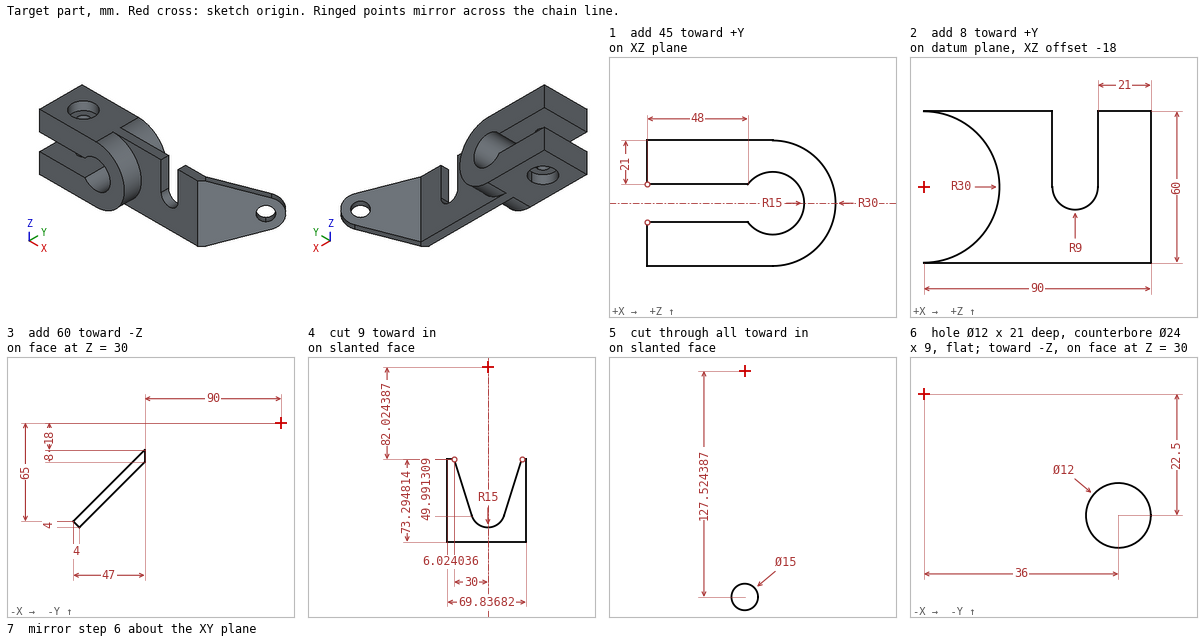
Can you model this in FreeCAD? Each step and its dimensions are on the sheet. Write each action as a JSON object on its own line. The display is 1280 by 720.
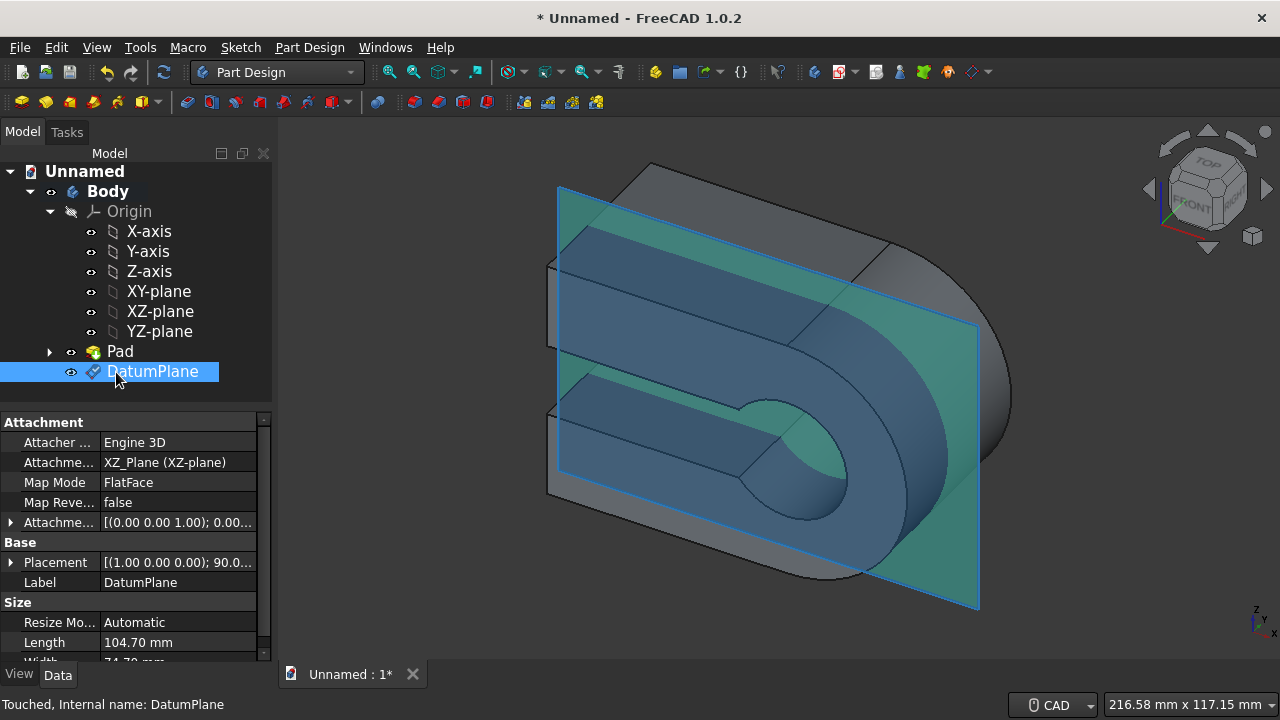
{"action": "left_click", "coordinate": [840, 72]}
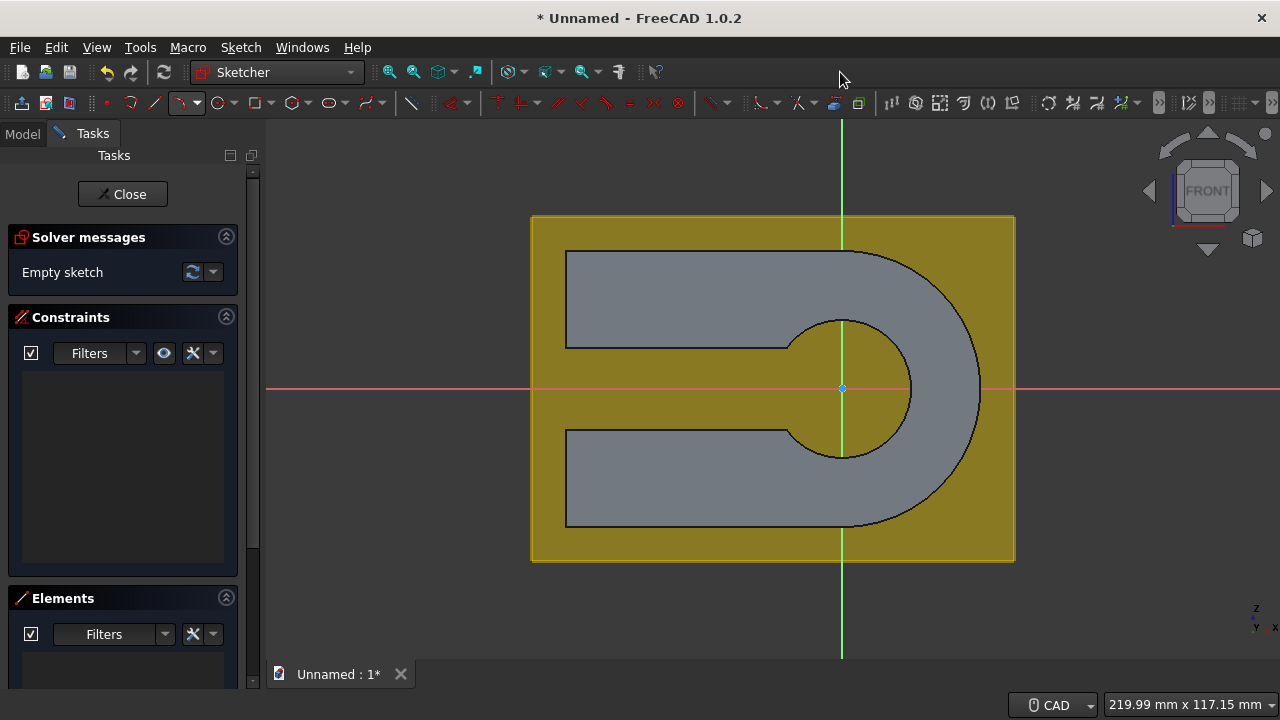
{"action": "left_click", "coordinate": [70, 104]}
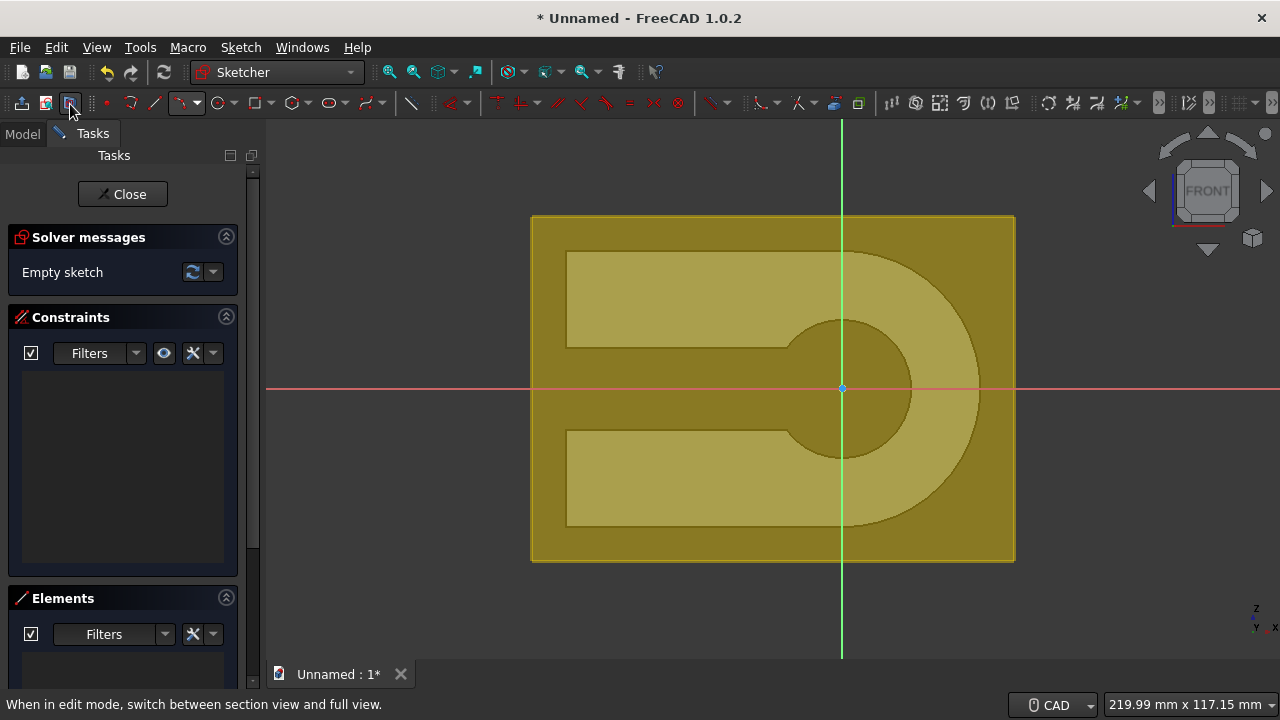
{"action": "scroll", "coordinate": [294, 389], "scroll_direction": "down", "scroll_amount": 1}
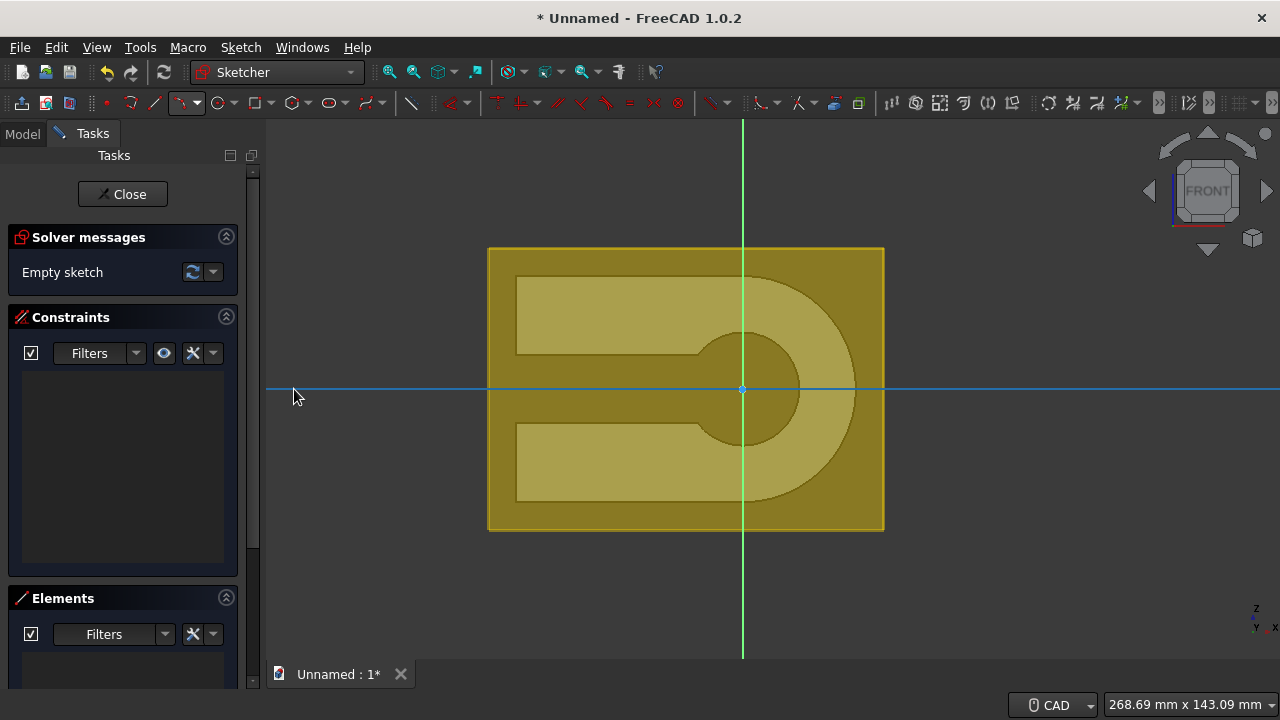
{"action": "scroll", "coordinate": [1115, 389], "scroll_direction": "up", "scroll_amount": 2}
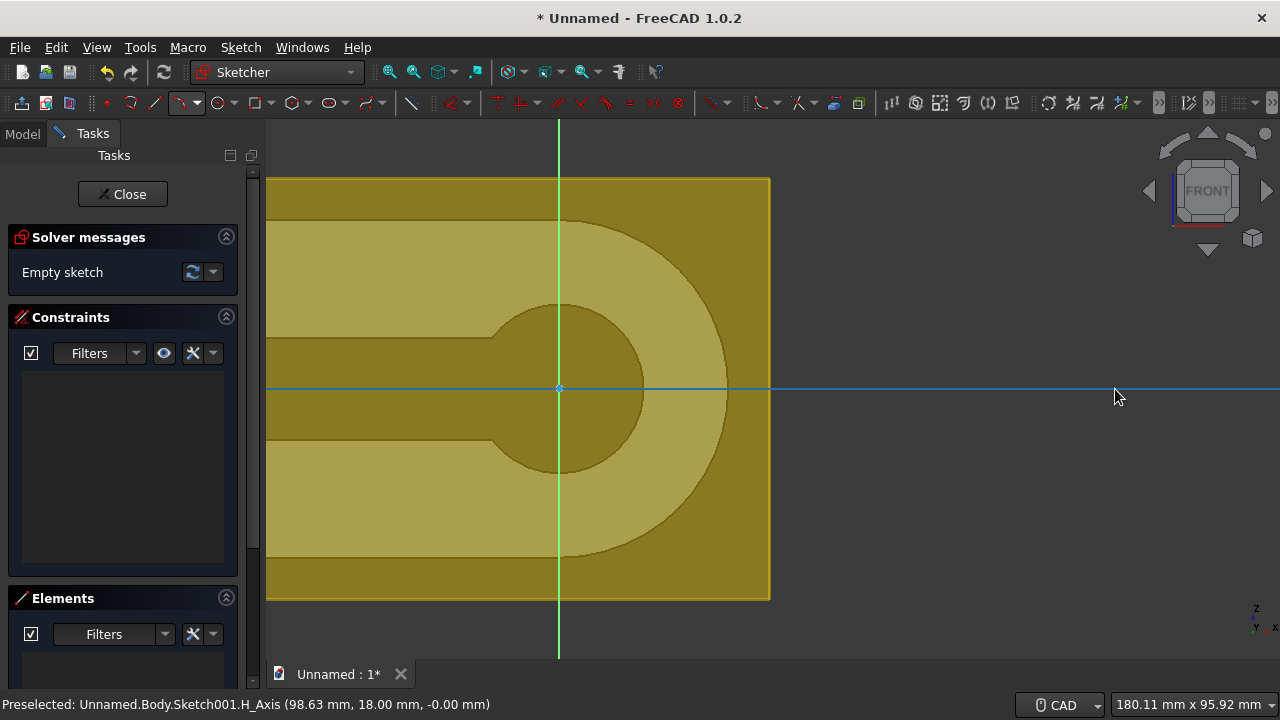
{"action": "left_click", "coordinate": [132, 104]}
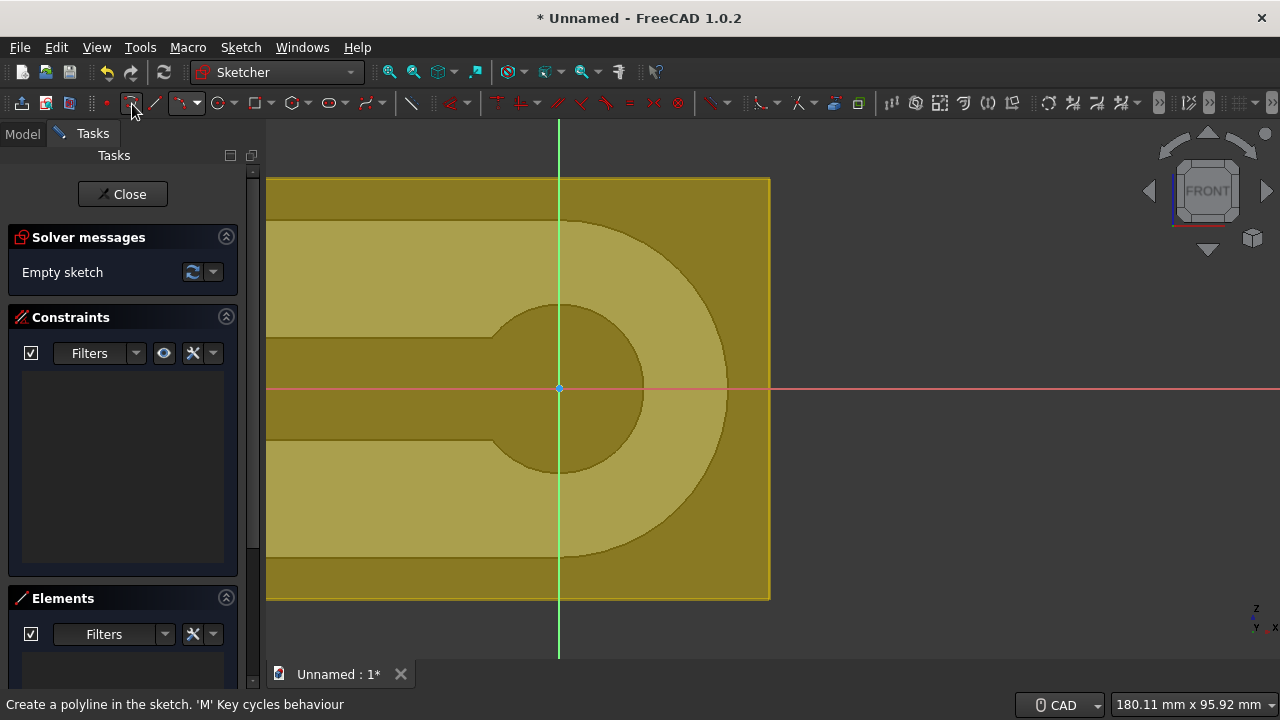
{"action": "left_click", "coordinate": [559, 558]}
{"action": "left_click", "coordinate": [1066, 558]}
{"action": "left_click", "coordinate": [1066, 220]}
{"action": "left_click", "coordinate": [948, 220]}
{"action": "left_click", "coordinate": [948, 389]}
{"action": "right_click", "coordinate": [948, 389]}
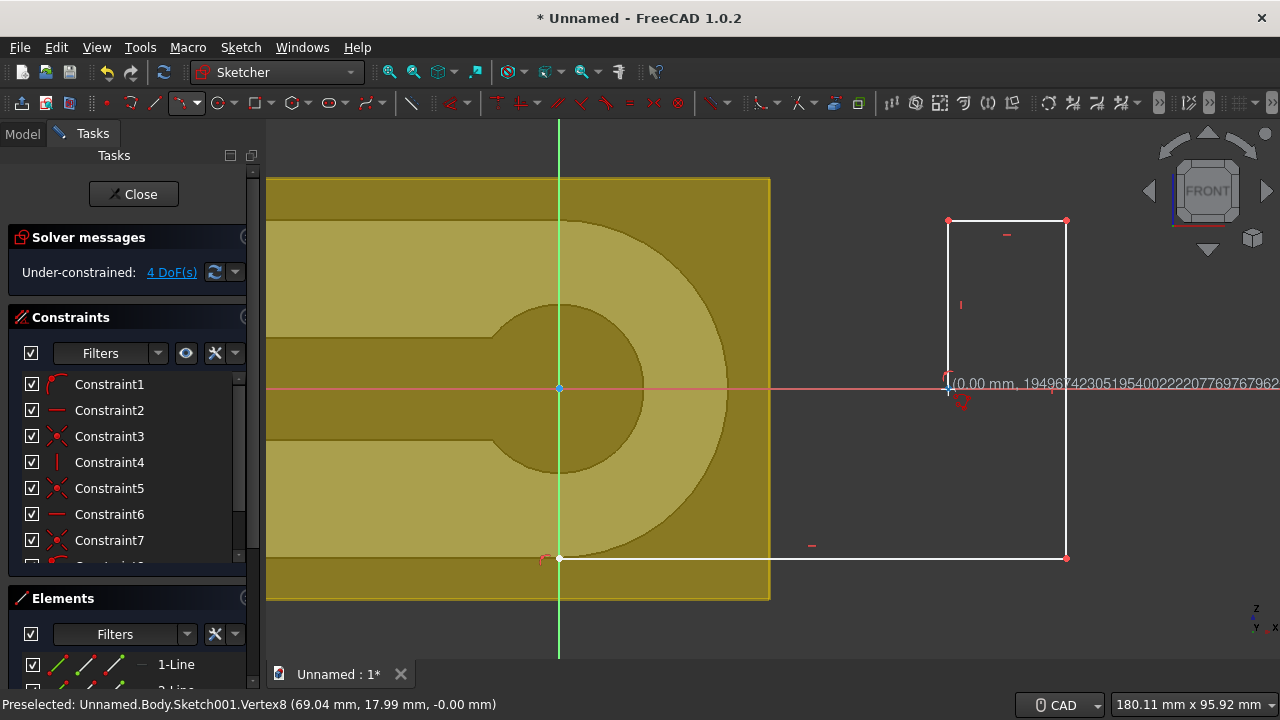
{"action": "left_click", "coordinate": [846, 389]}
{"action": "left_click", "coordinate": [846, 220]}
{"action": "left_click", "coordinate": [559, 220]}
{"action": "right_click", "coordinate": [559, 220]}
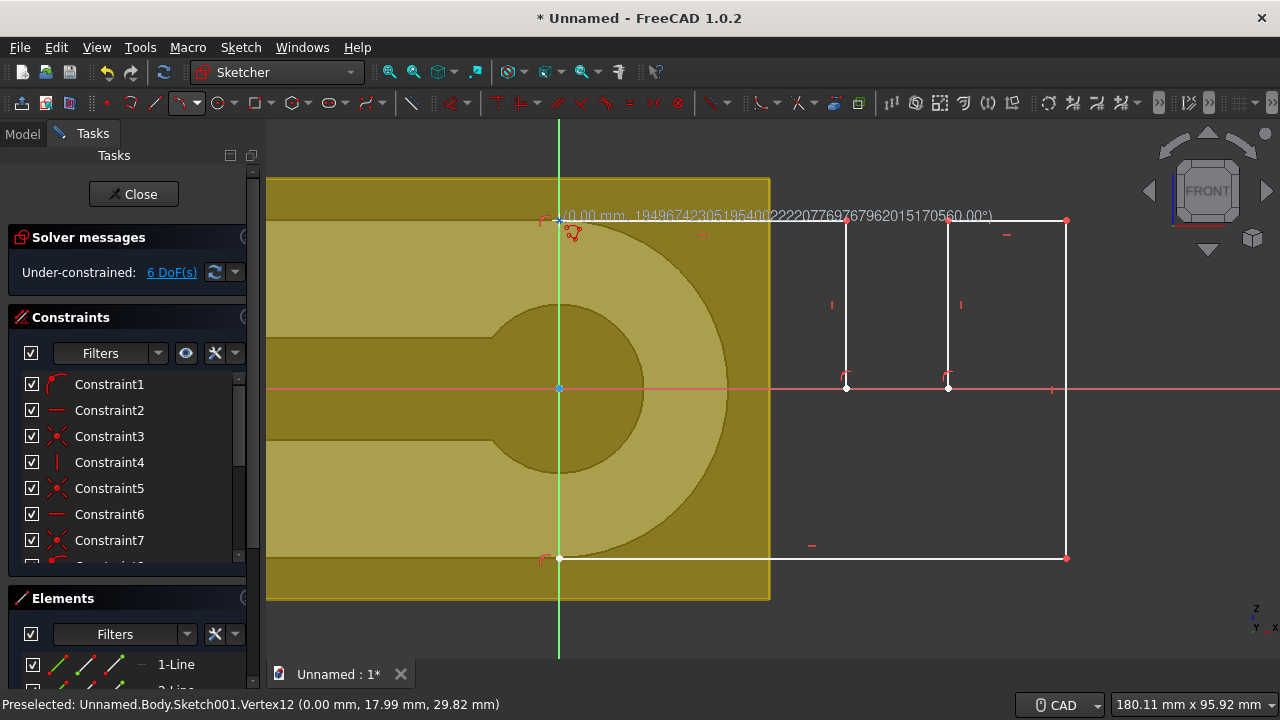
{"action": "key", "text": "g 3 a"}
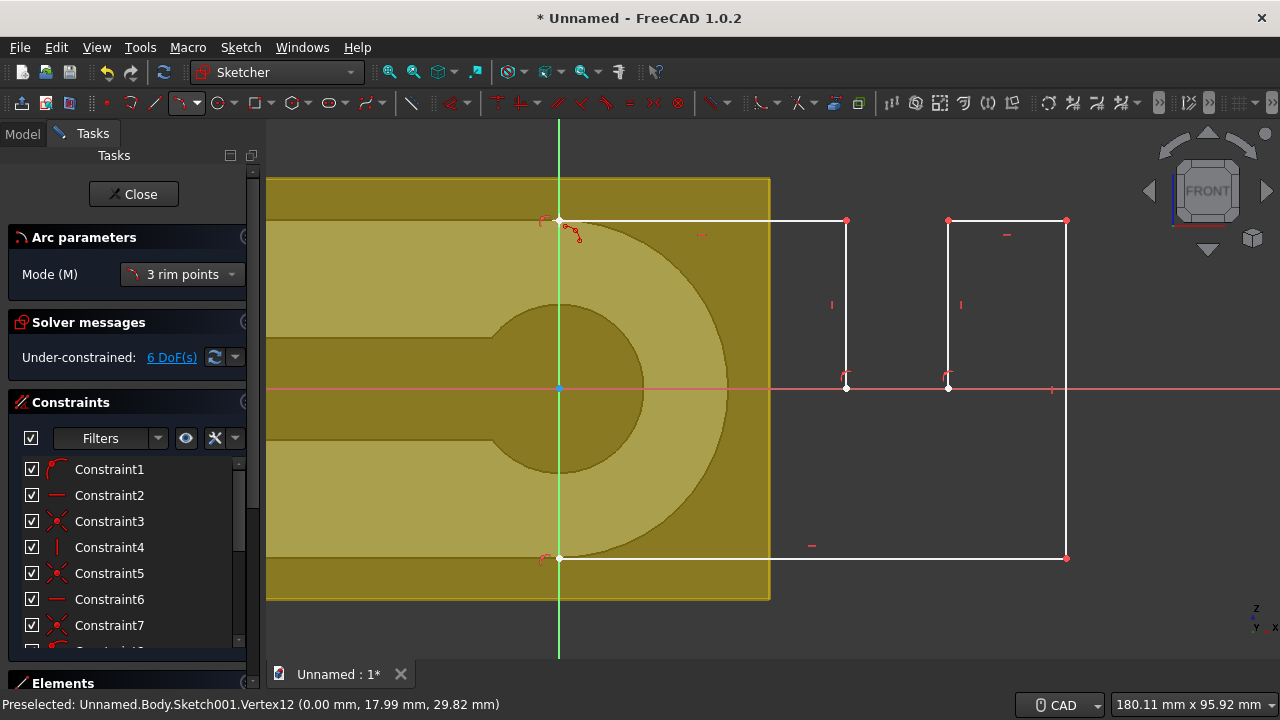
{"action": "left_click", "coordinate": [948, 389]}
{"action": "left_click", "coordinate": [846, 389]}
{"action": "left_click", "coordinate": [897, 440]}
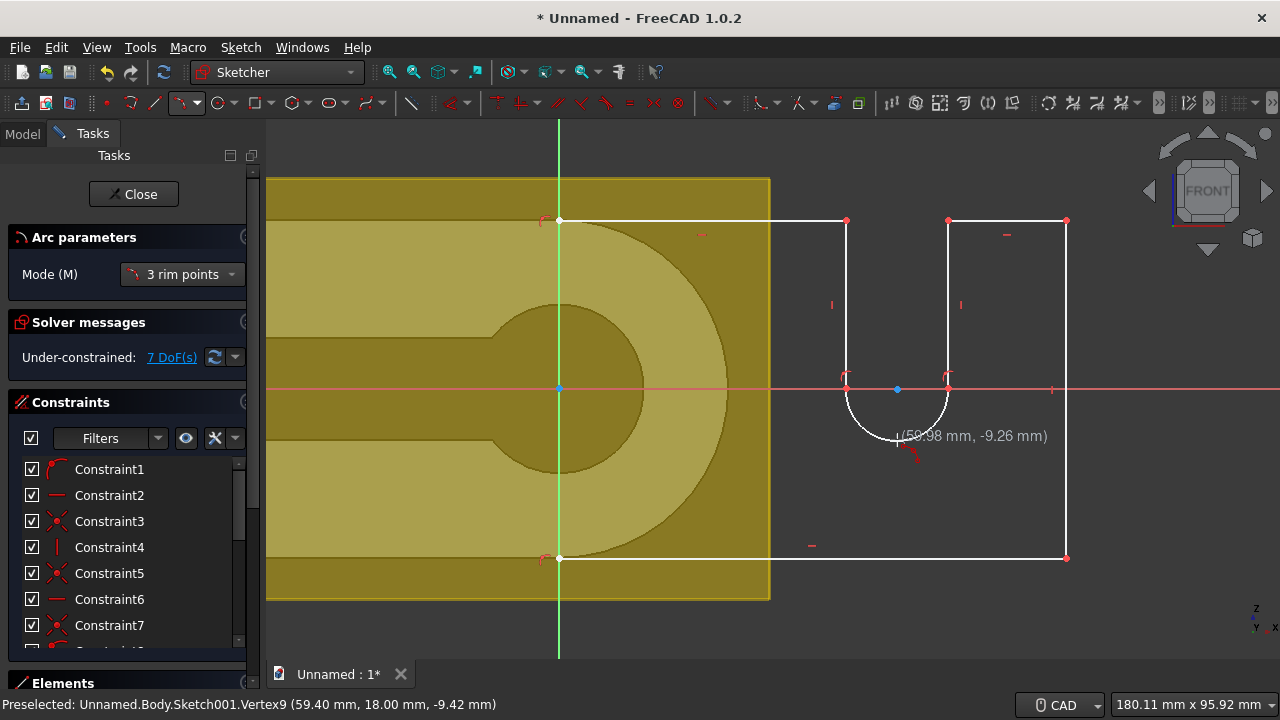
{"action": "left_click", "coordinate": [559, 221]}
{"action": "left_click", "coordinate": [559, 559]}
{"action": "left_click", "coordinate": [720, 441]}
{"action": "key", "text": "Escape"}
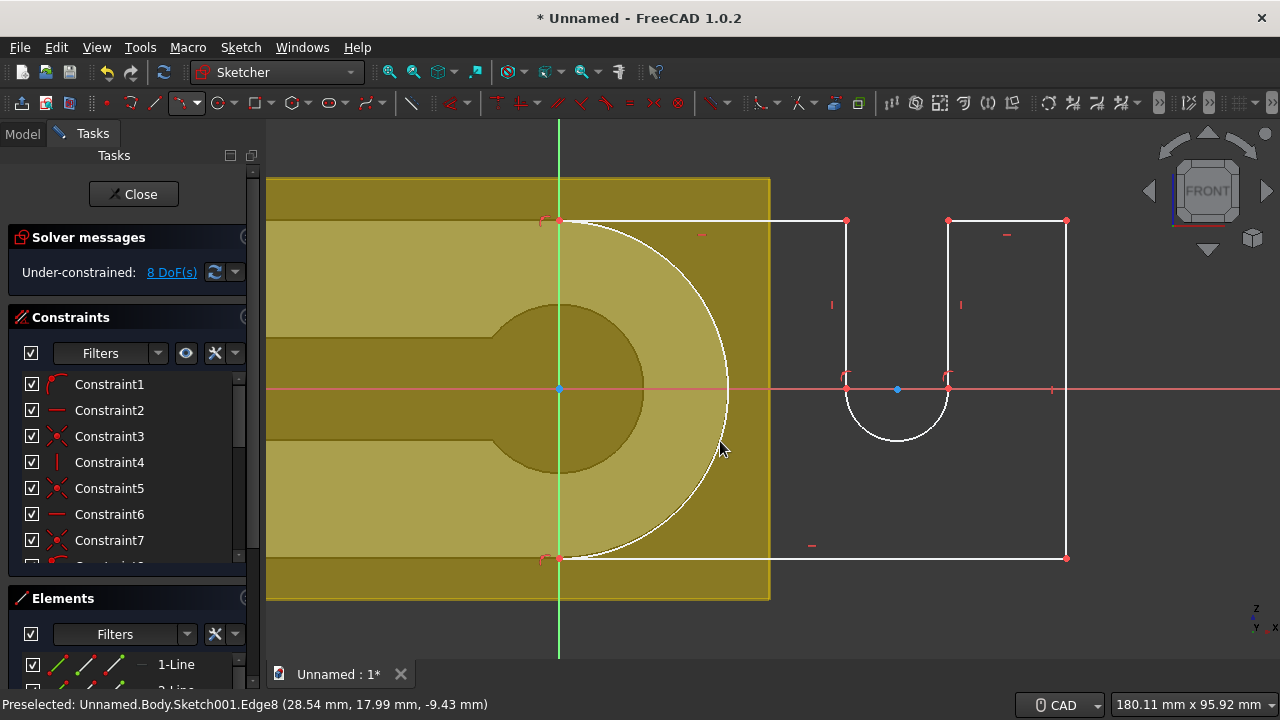
{"action": "left_click", "coordinate": [948, 271]}